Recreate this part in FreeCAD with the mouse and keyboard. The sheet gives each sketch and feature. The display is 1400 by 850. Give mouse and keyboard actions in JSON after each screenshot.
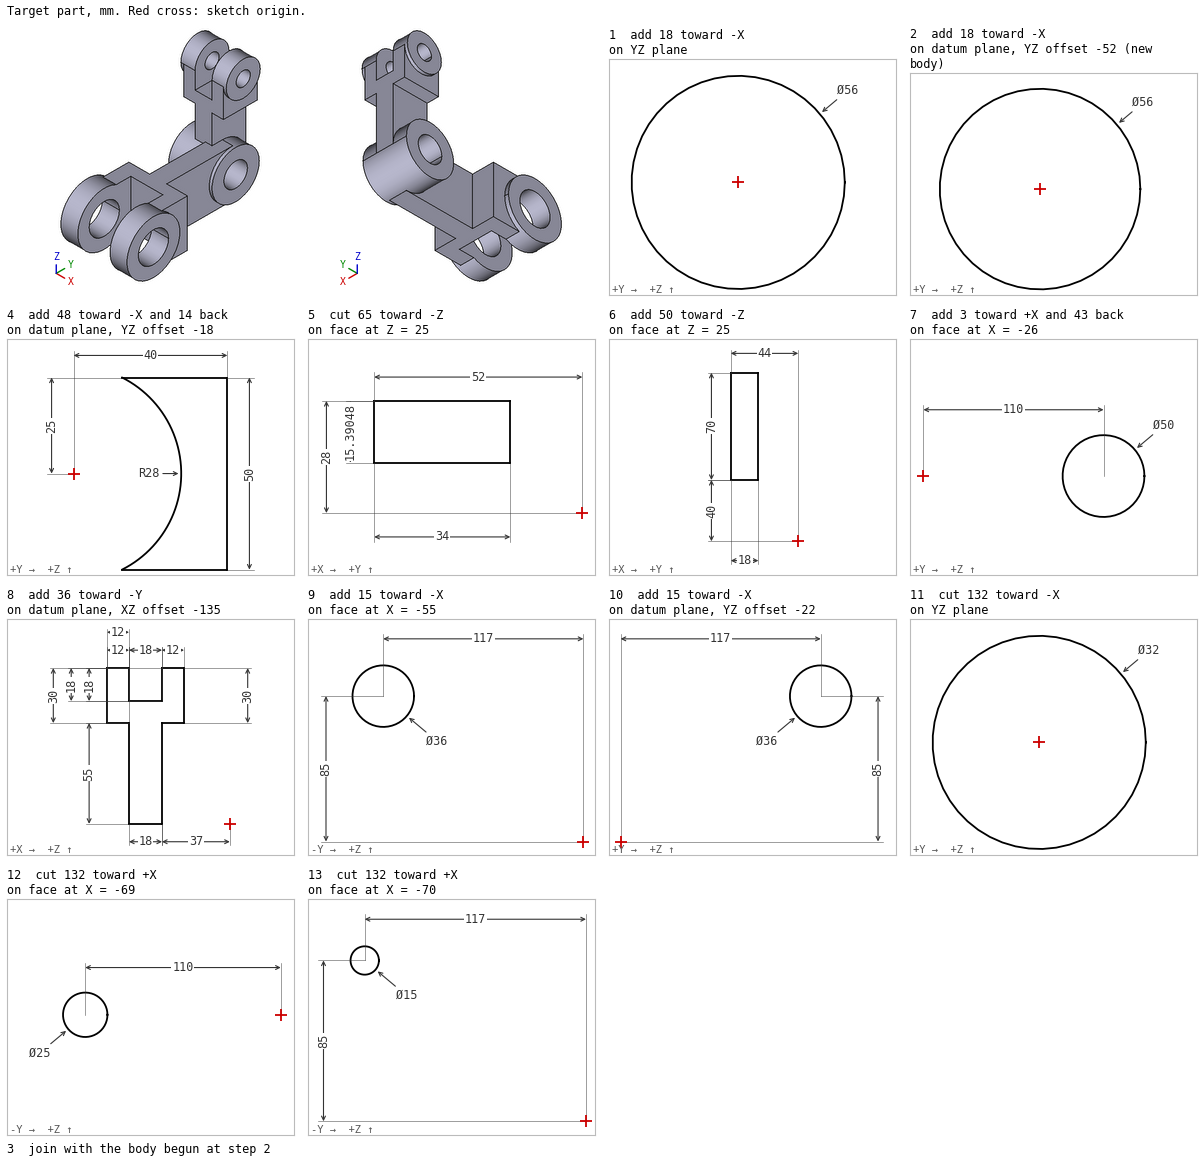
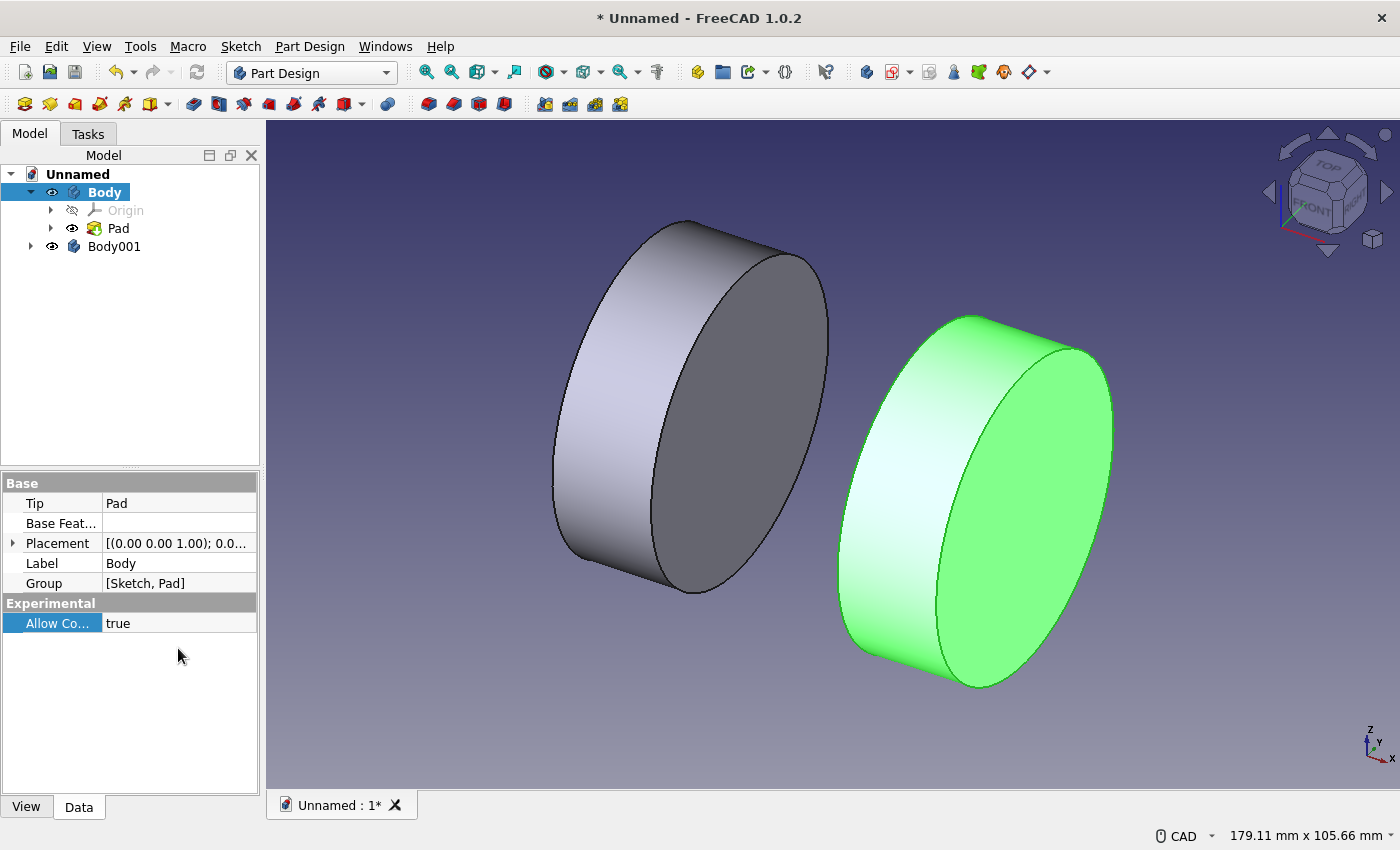
{"action": "left_click", "coordinate": [97, 246]}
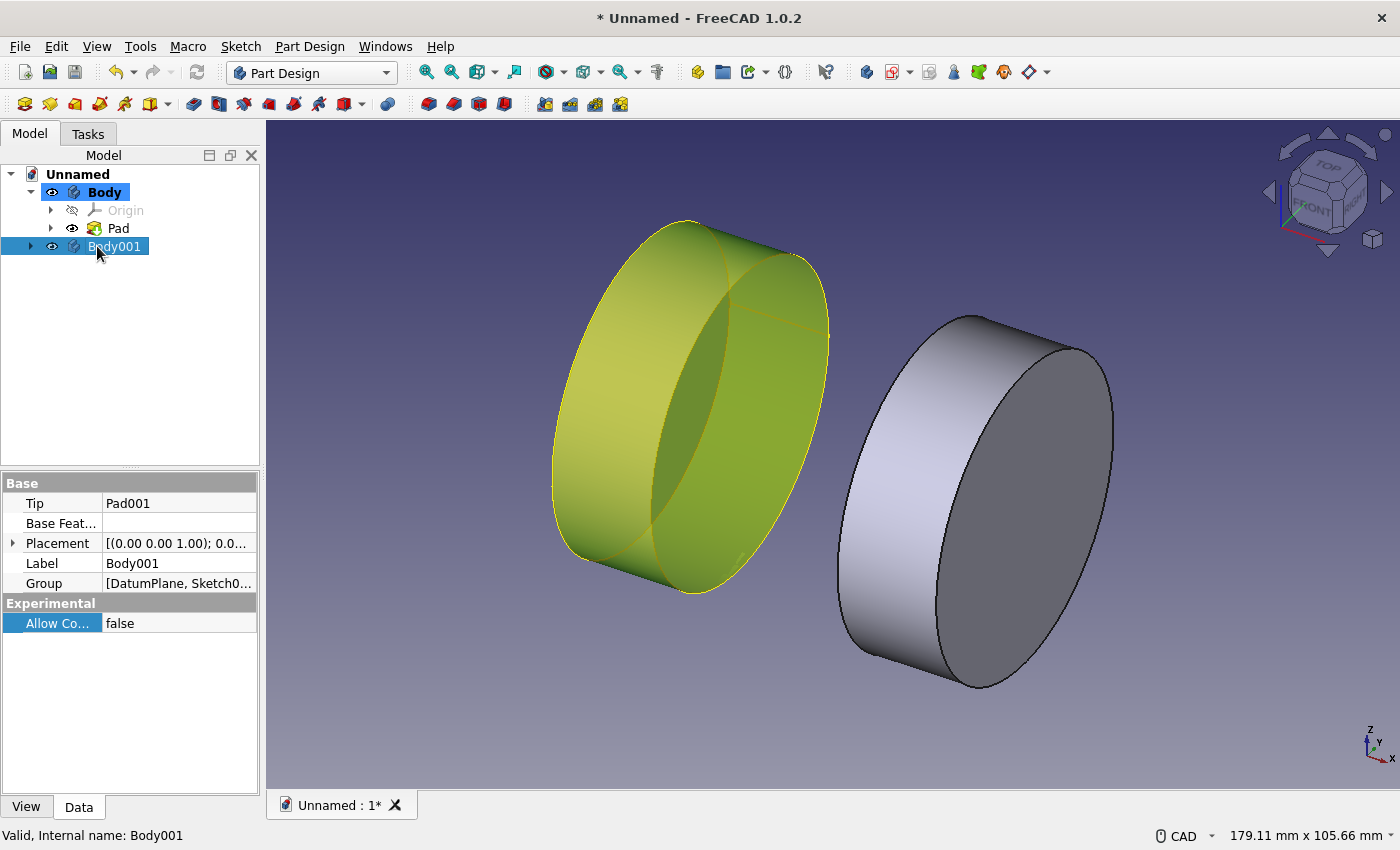
{"action": "left_click", "coordinate": [388, 104]}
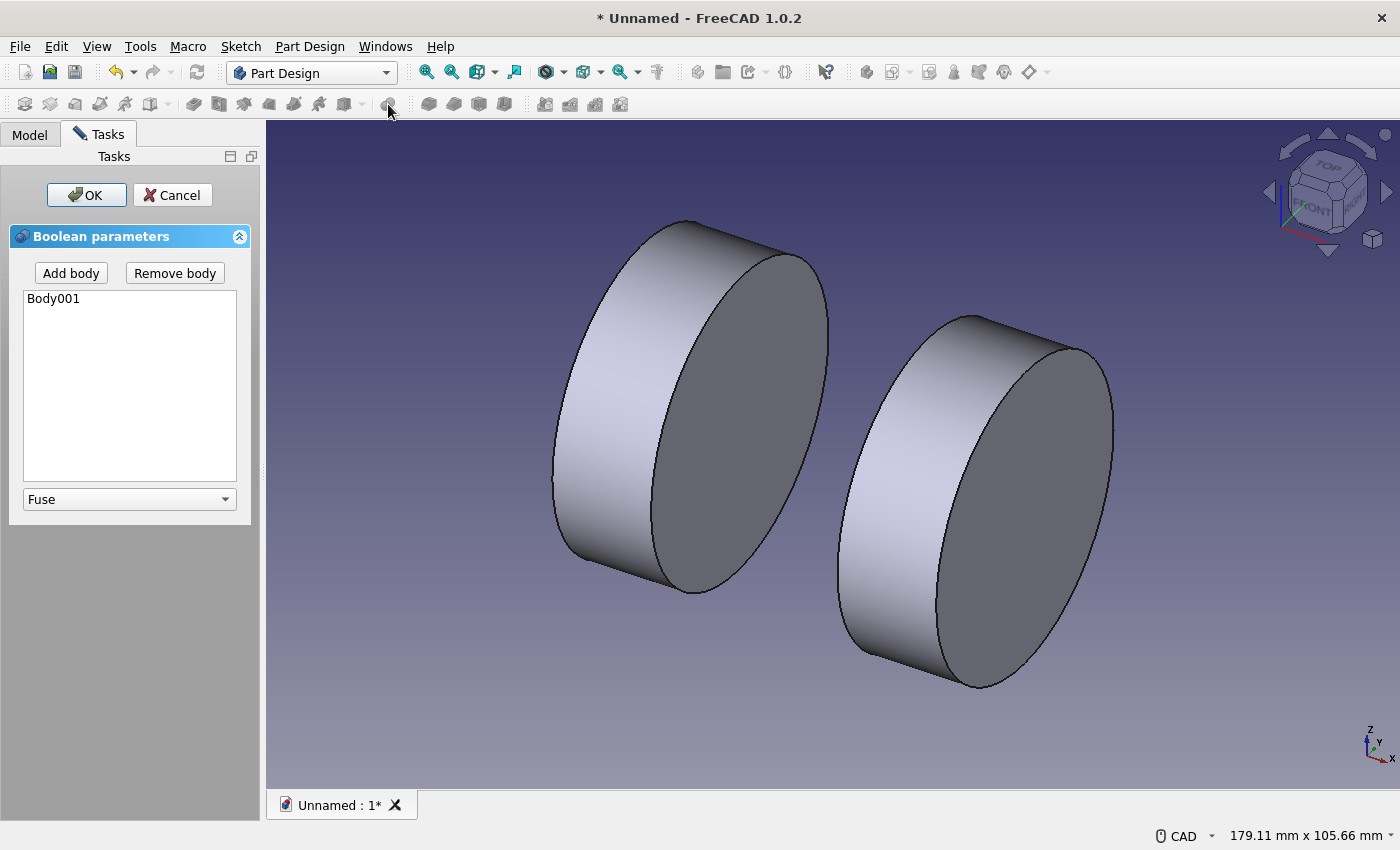
{"action": "left_click", "coordinate": [87, 195]}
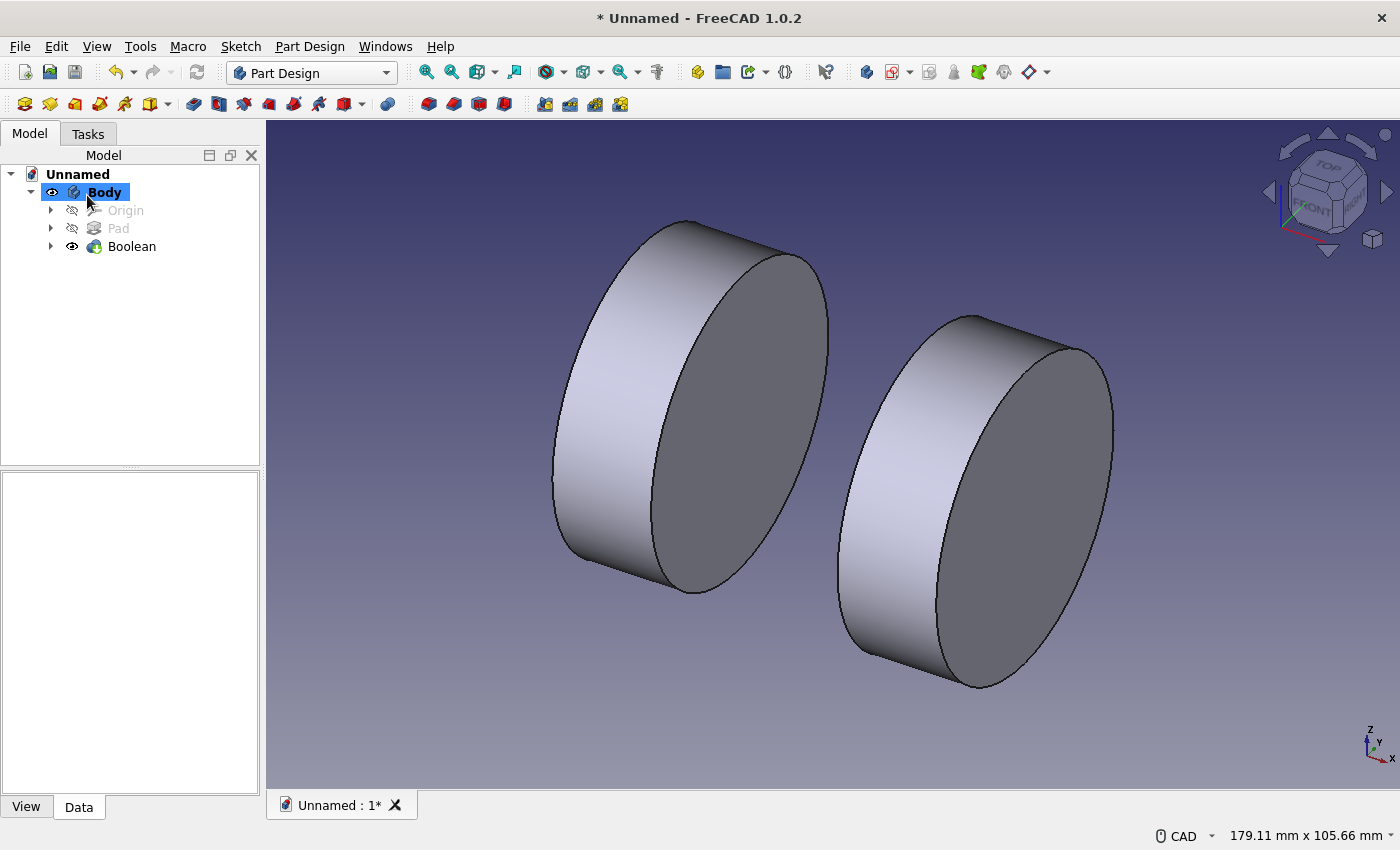
{"action": "left_click", "coordinate": [51, 210]}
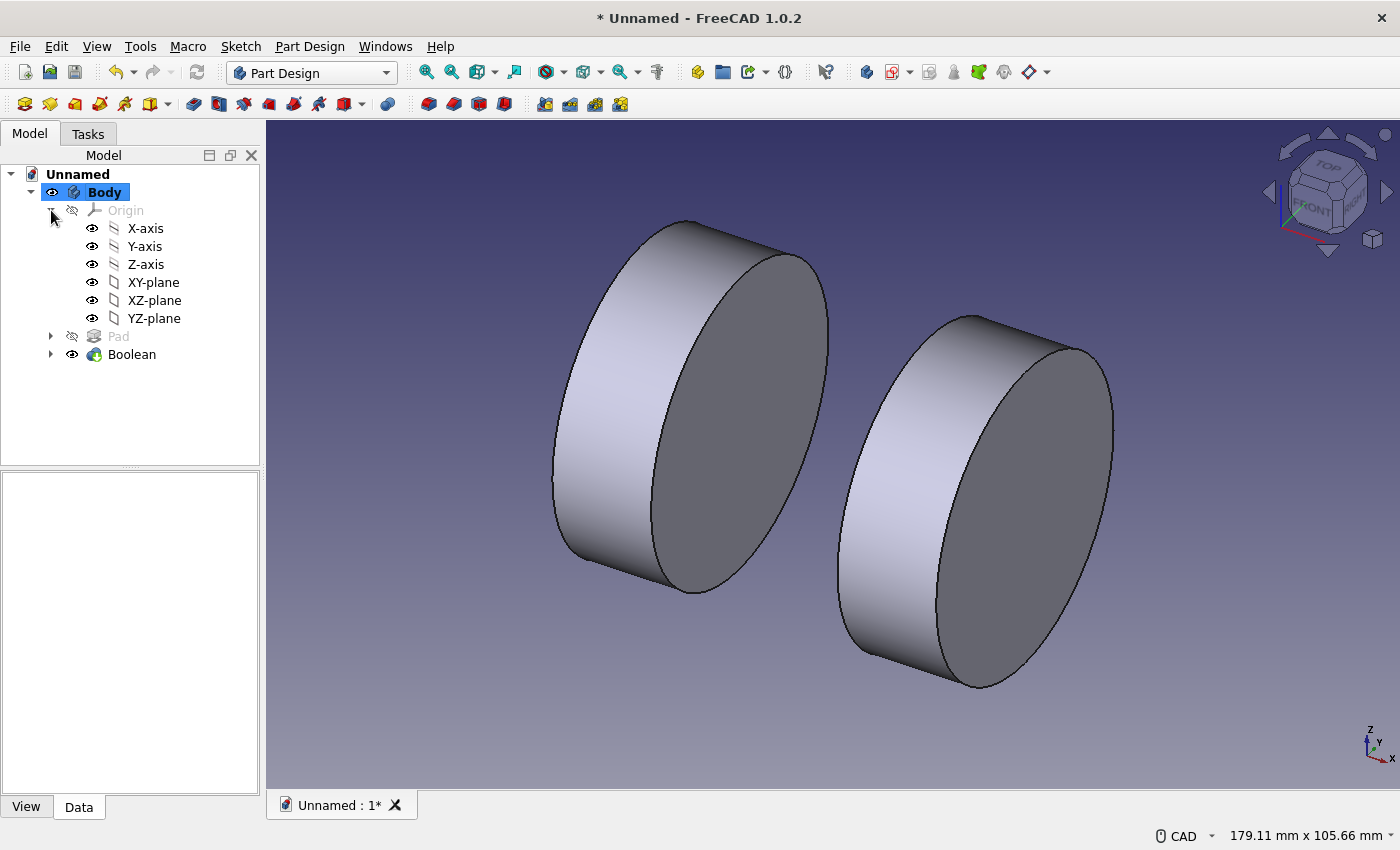
{"action": "left_click", "coordinate": [137, 318]}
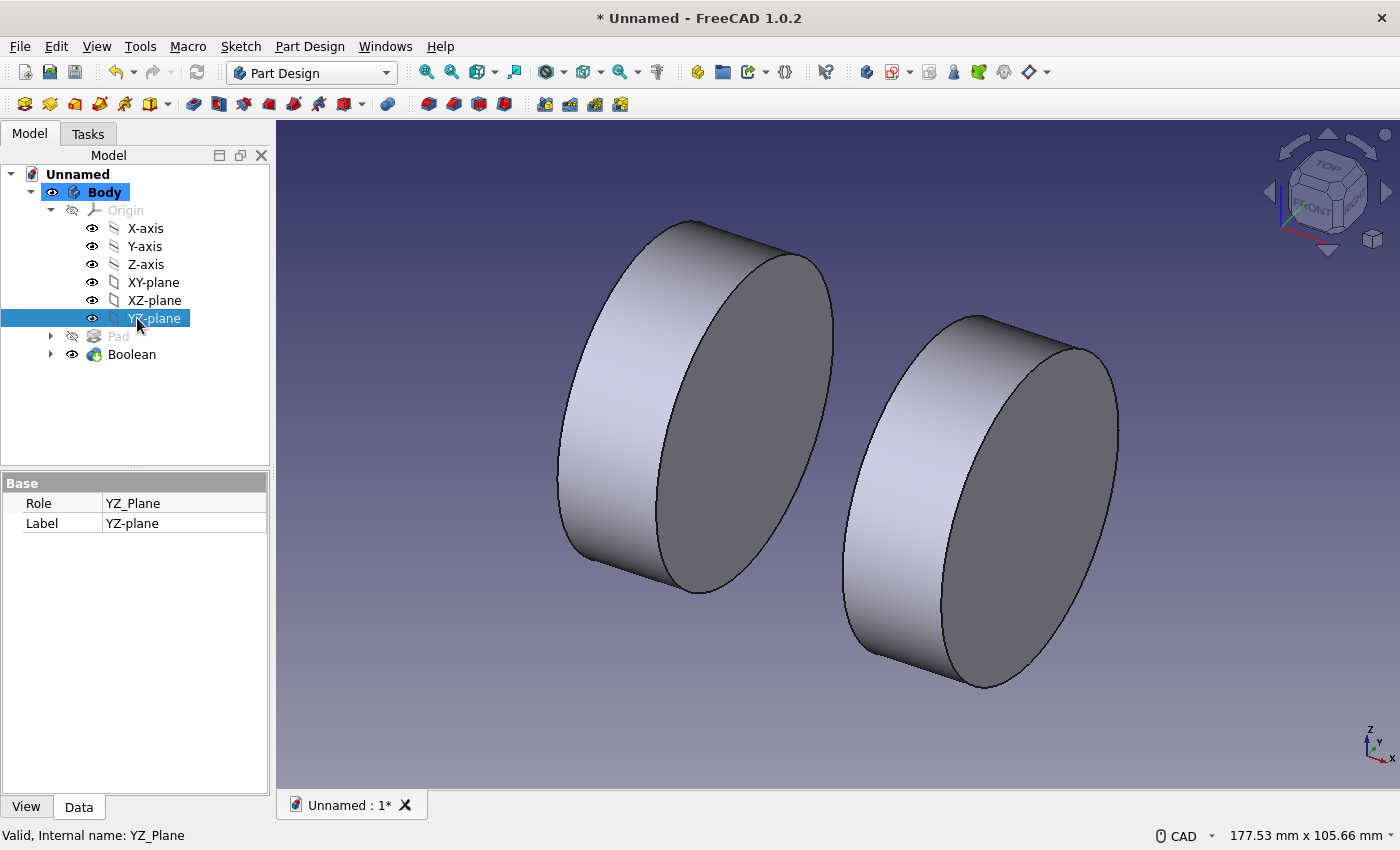
{"action": "left_click", "coordinate": [1028, 72]}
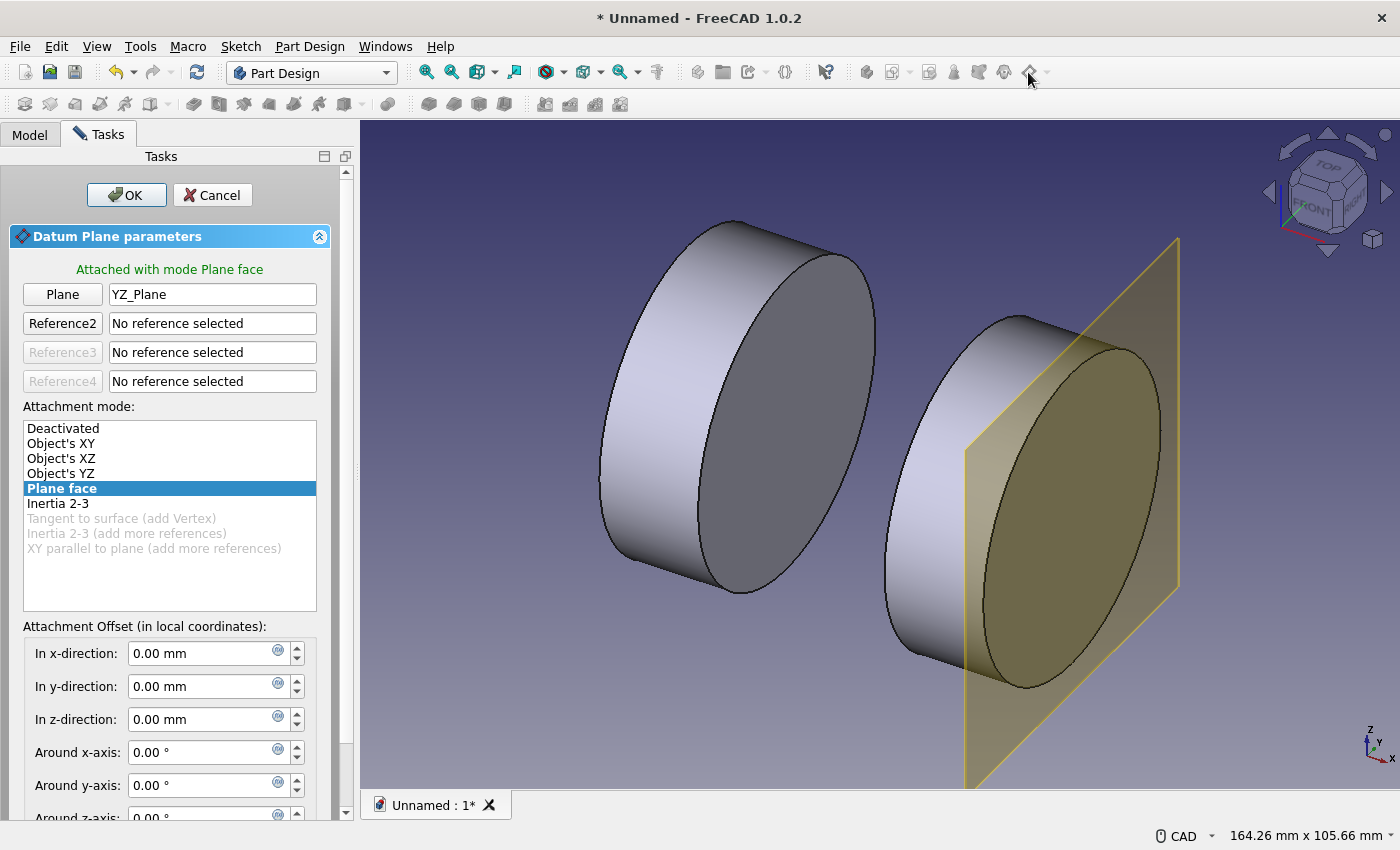
{"action": "triple_click", "coordinate": [210, 720]}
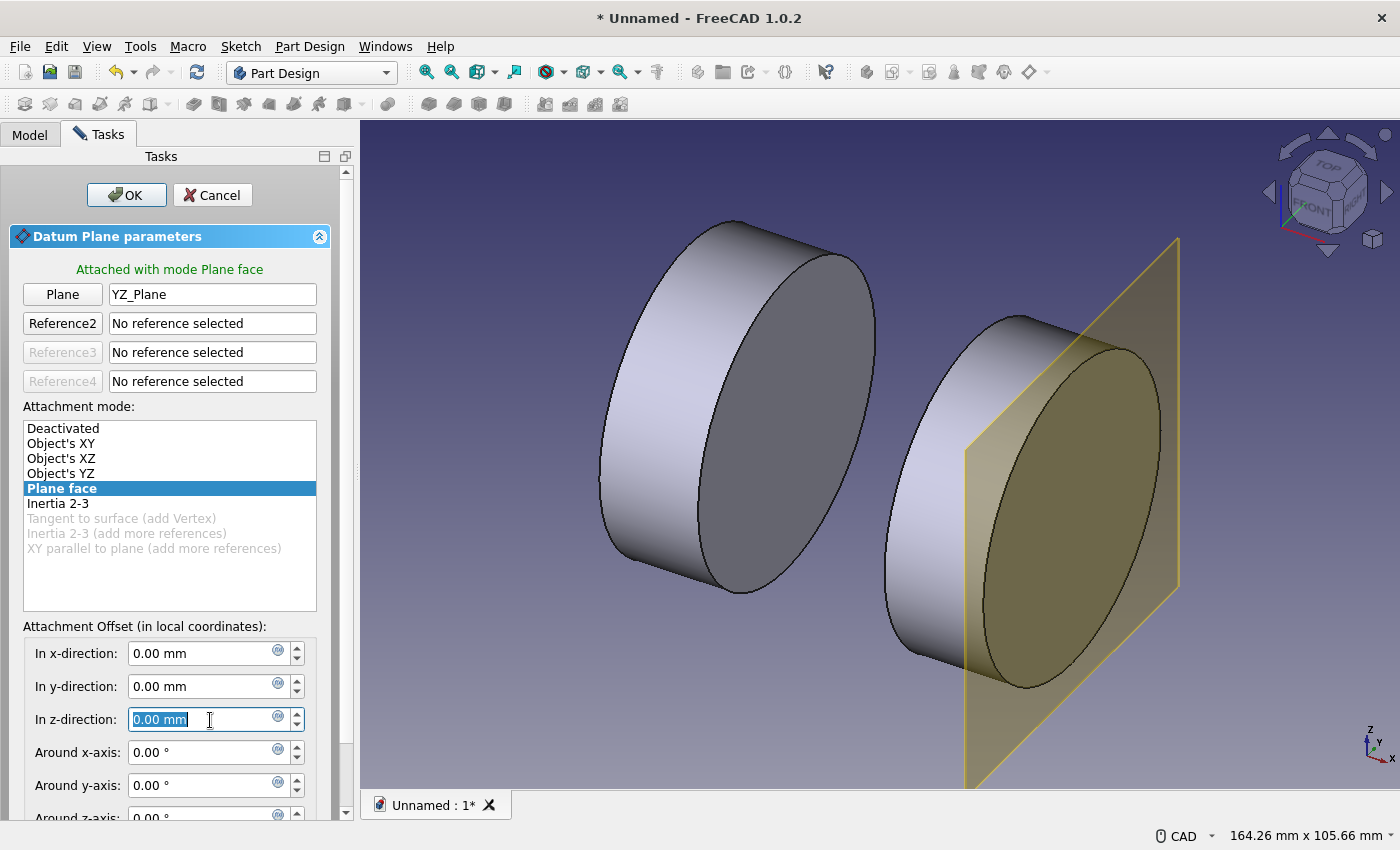
{"action": "type", "text": "-18"}
{"action": "key", "text": "Tab"}